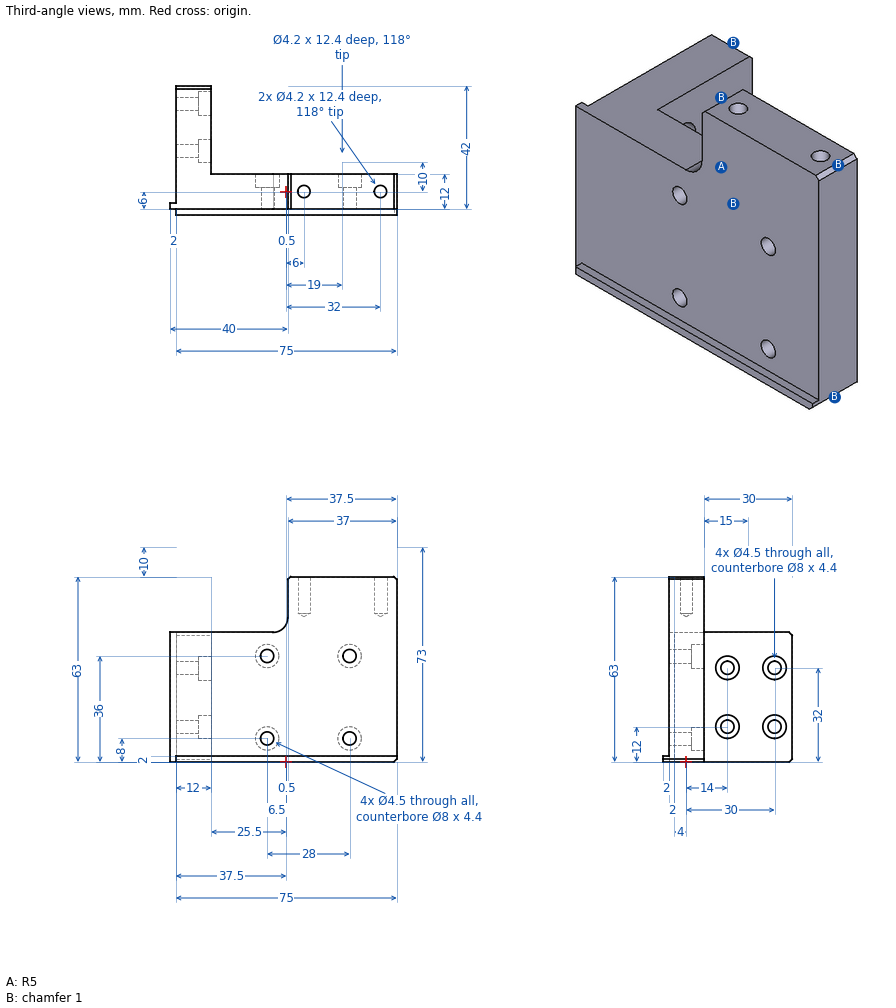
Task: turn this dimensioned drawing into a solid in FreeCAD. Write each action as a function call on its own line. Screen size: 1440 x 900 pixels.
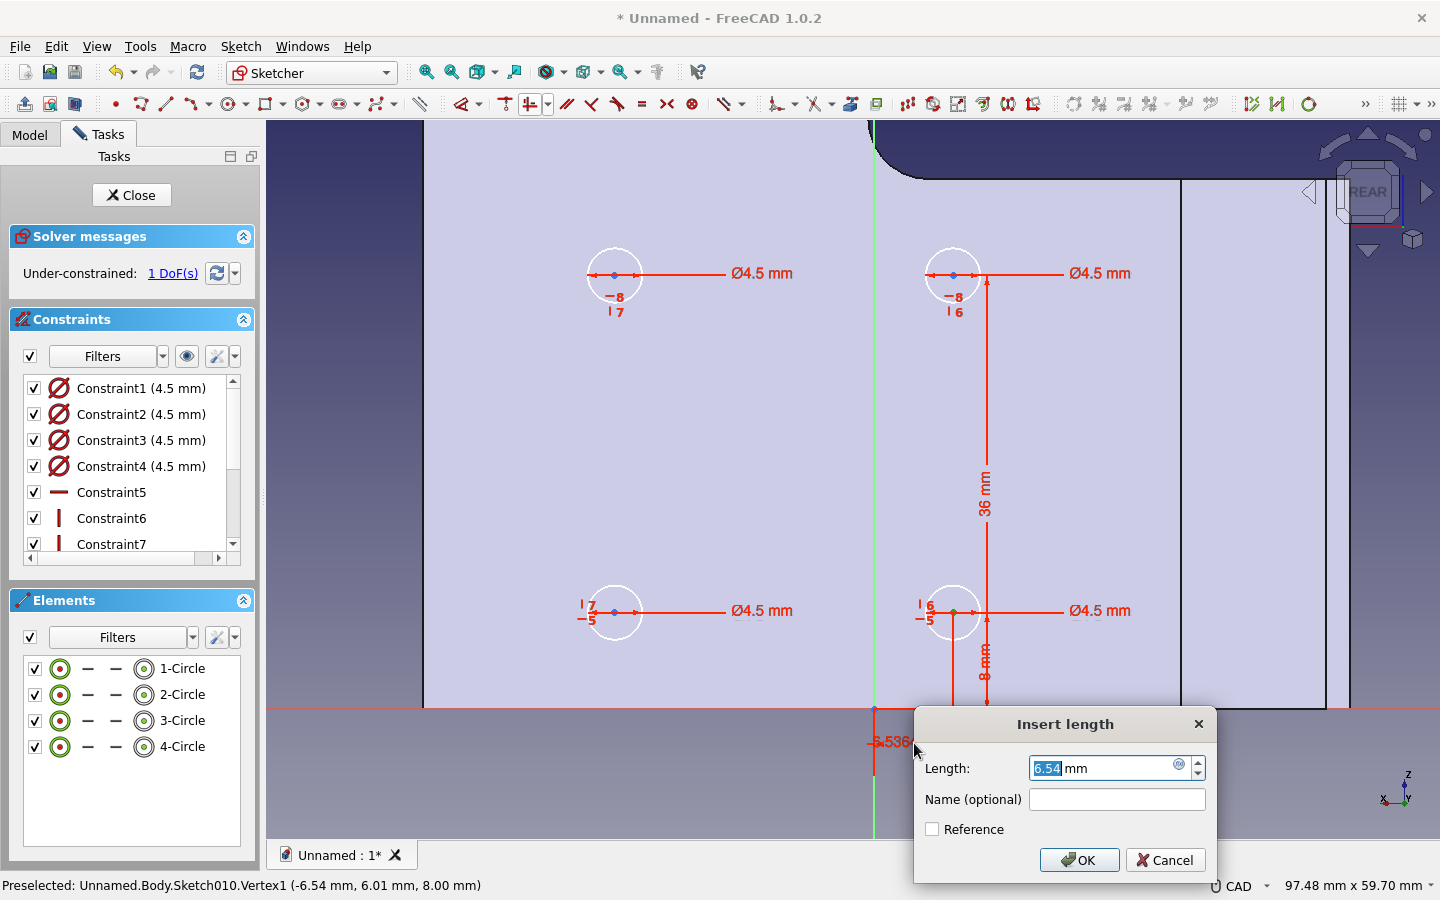
text(6.5)
key(Return)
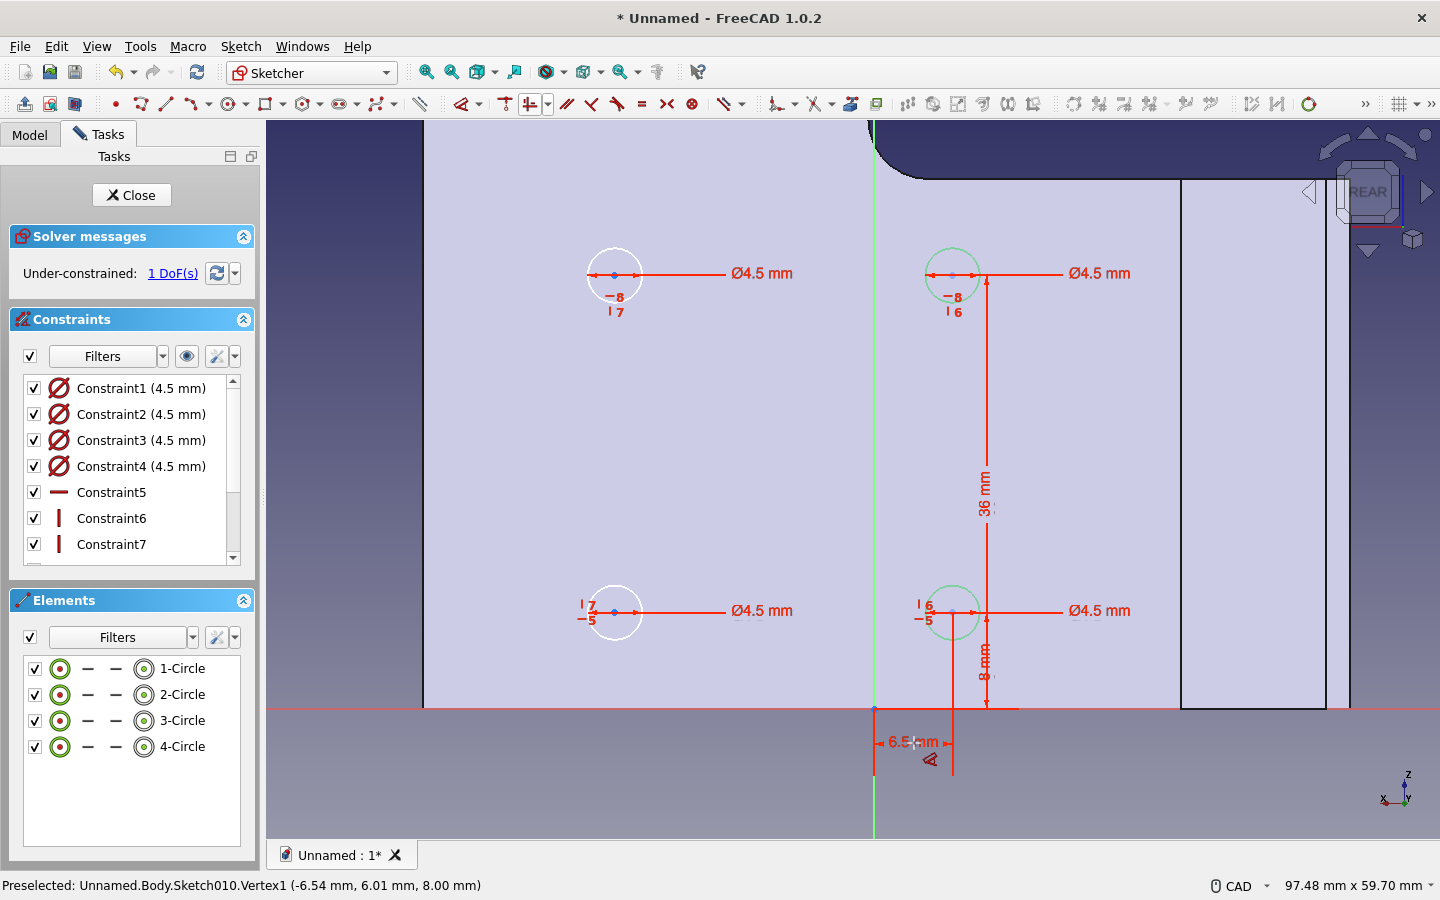
click(953, 613)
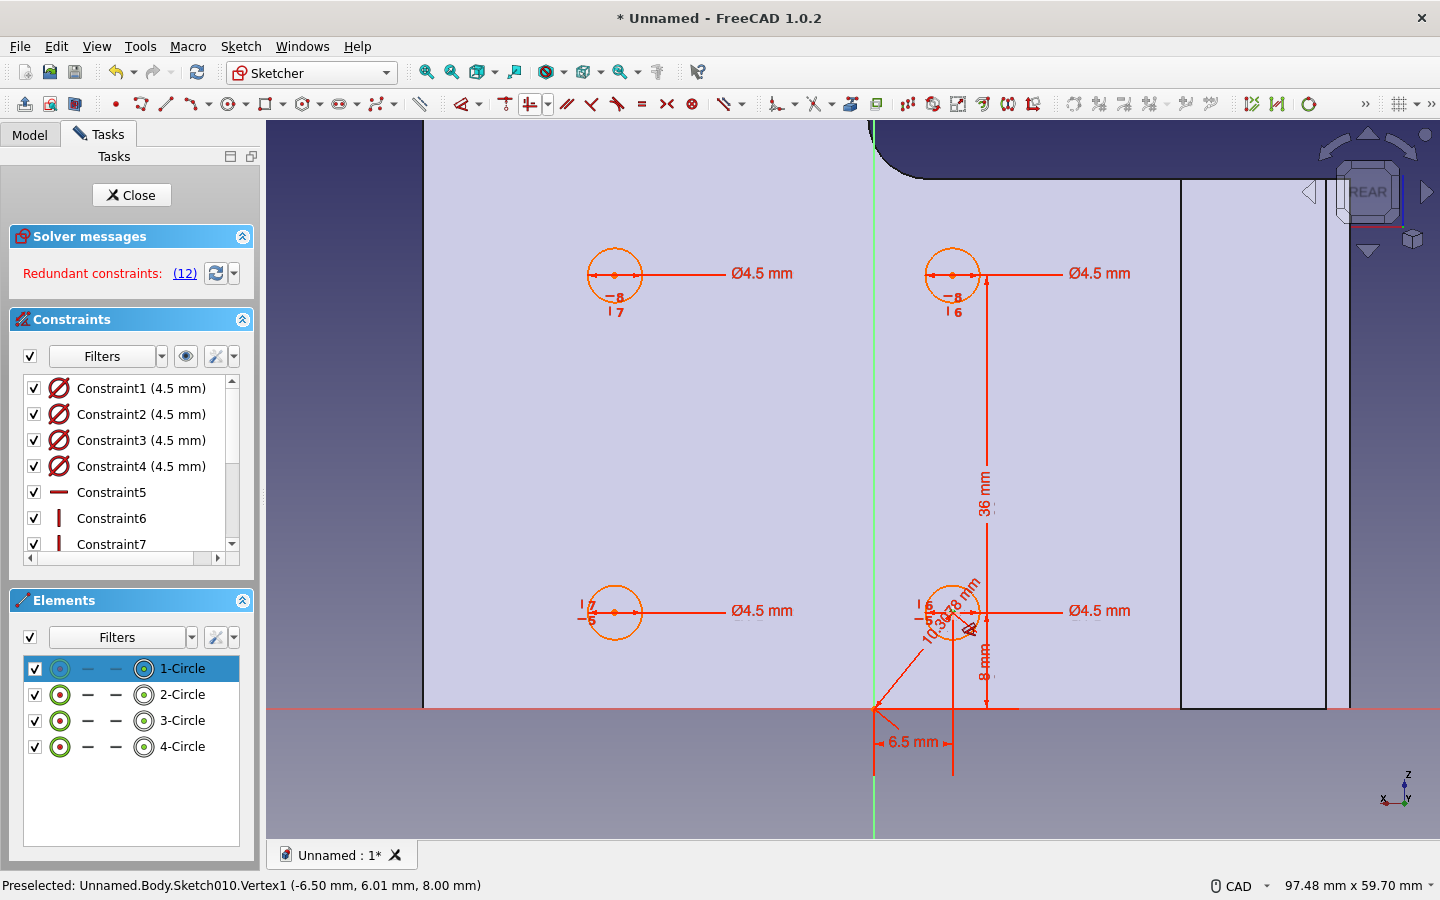
click(615, 613)
click(784, 647)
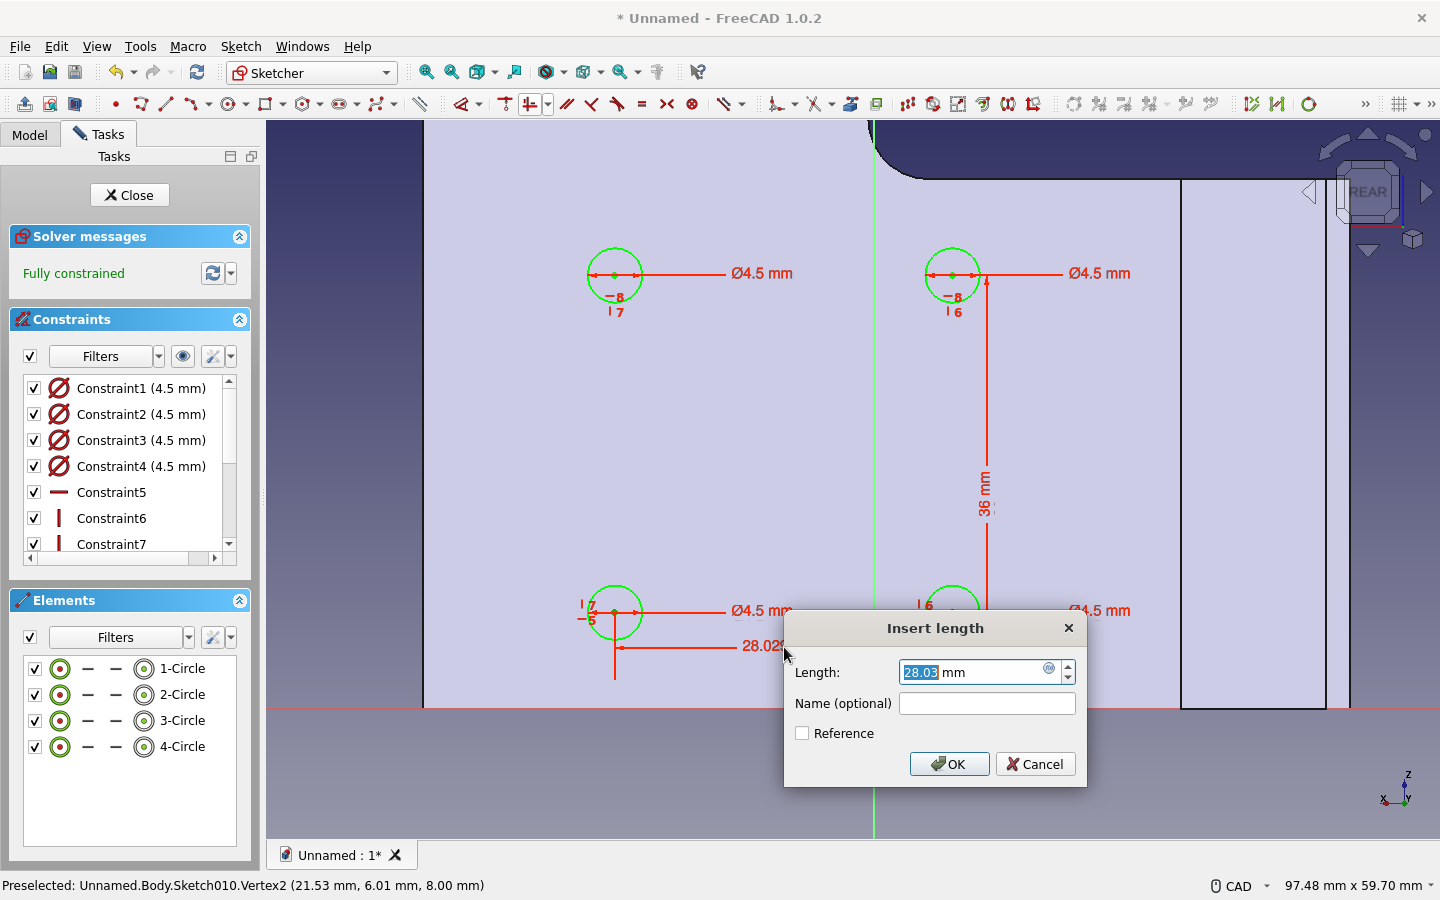
text(28)
key(Return)
key(Escape)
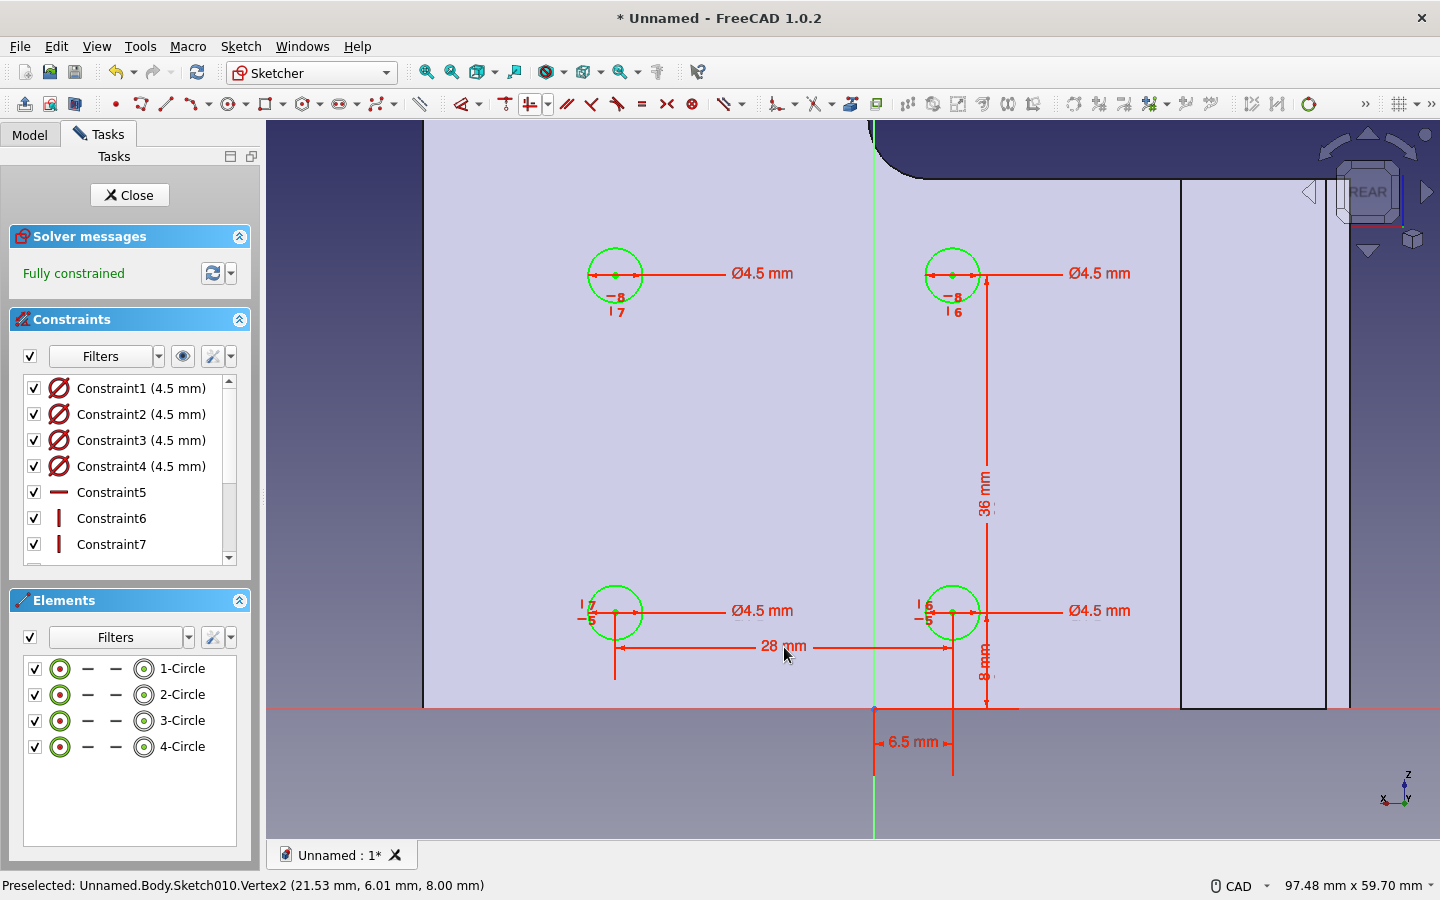
click(130, 195)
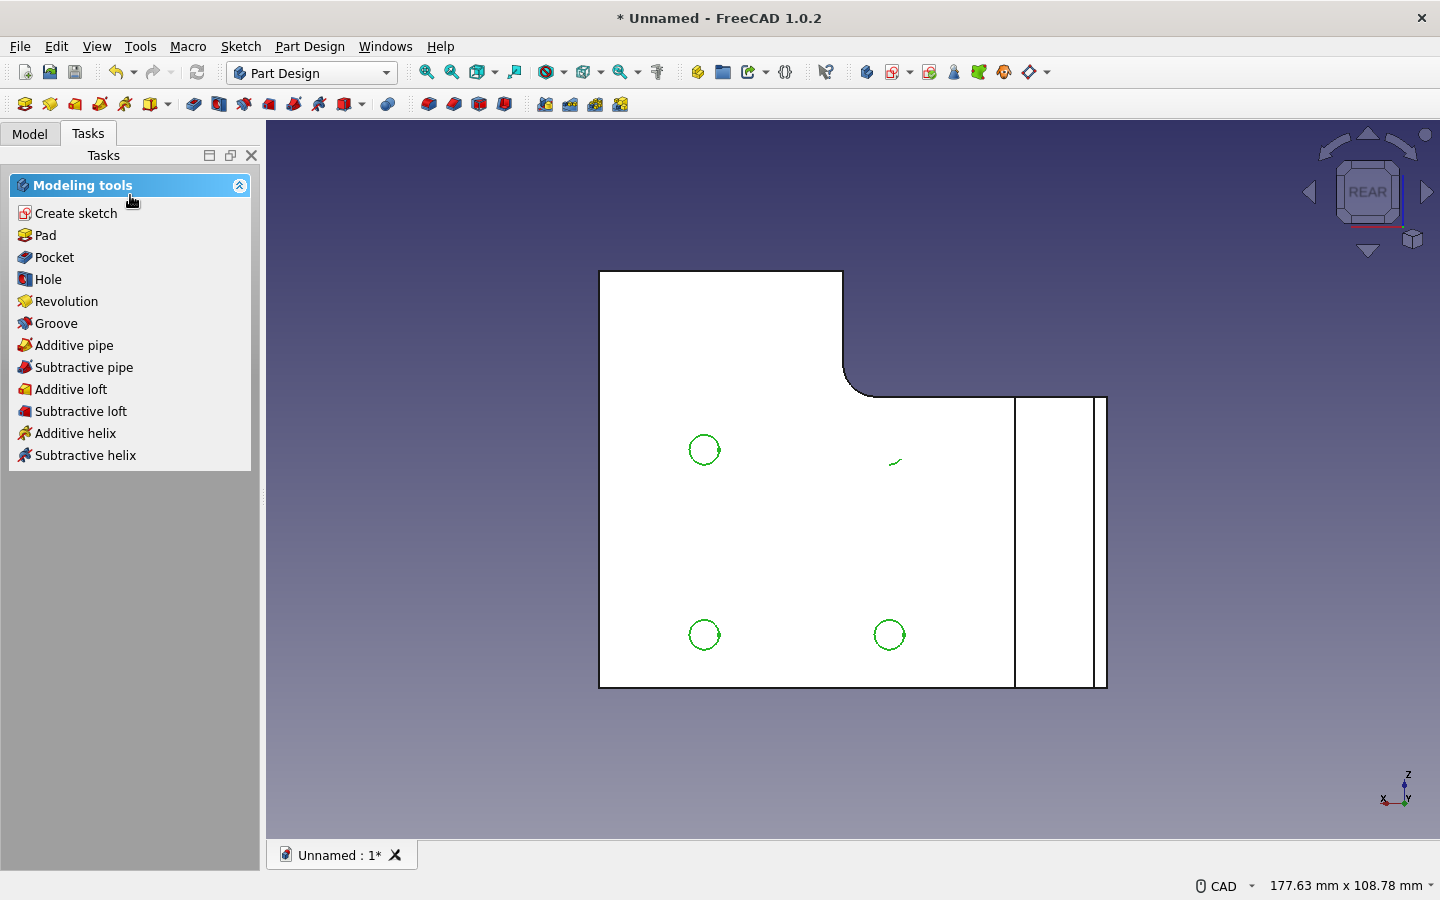
click(219, 104)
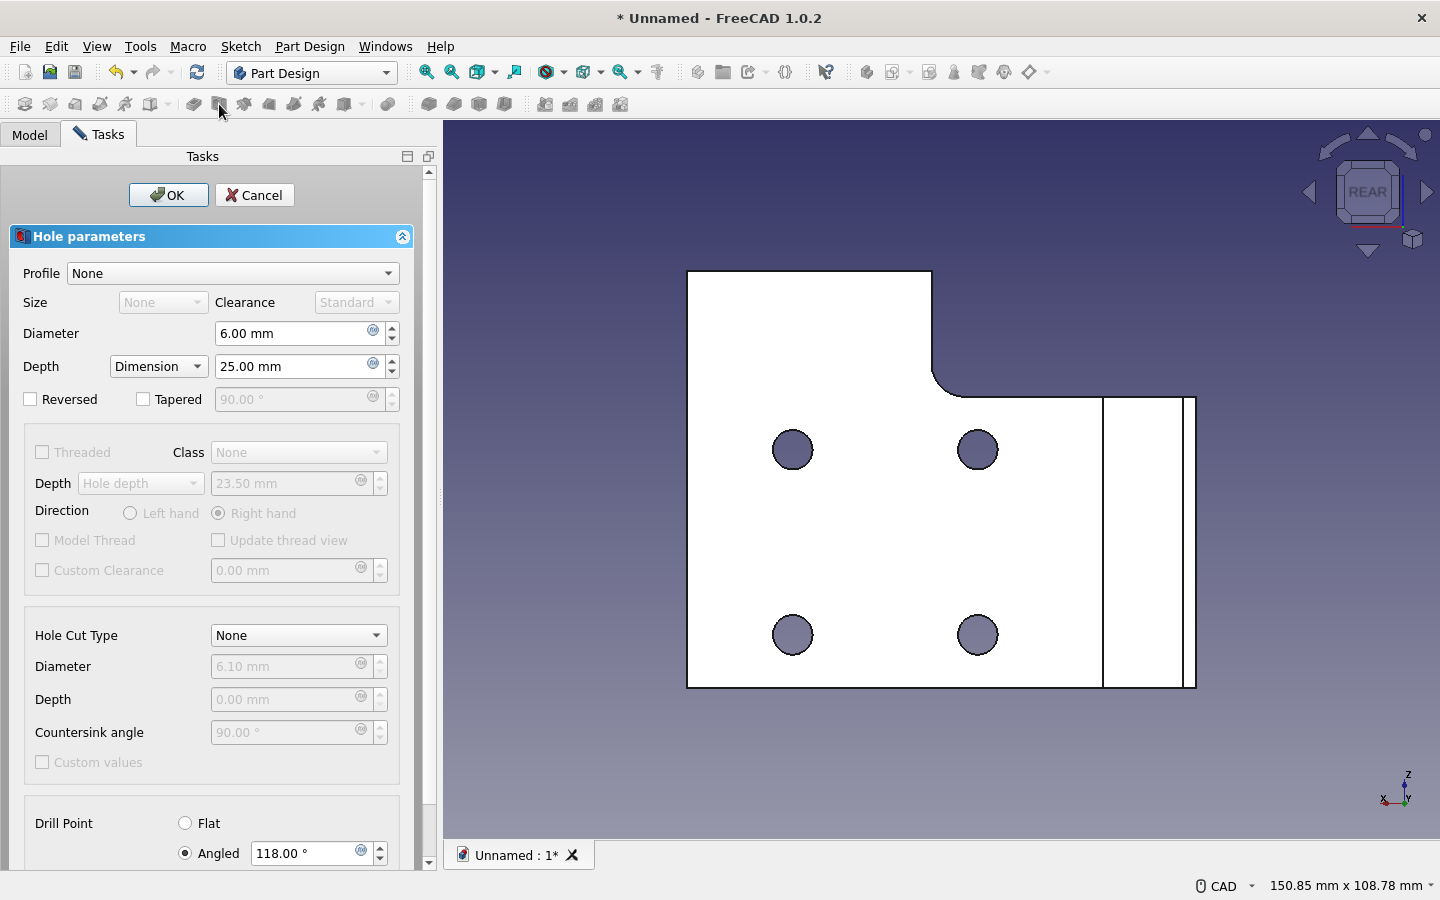
triple_click(300, 334)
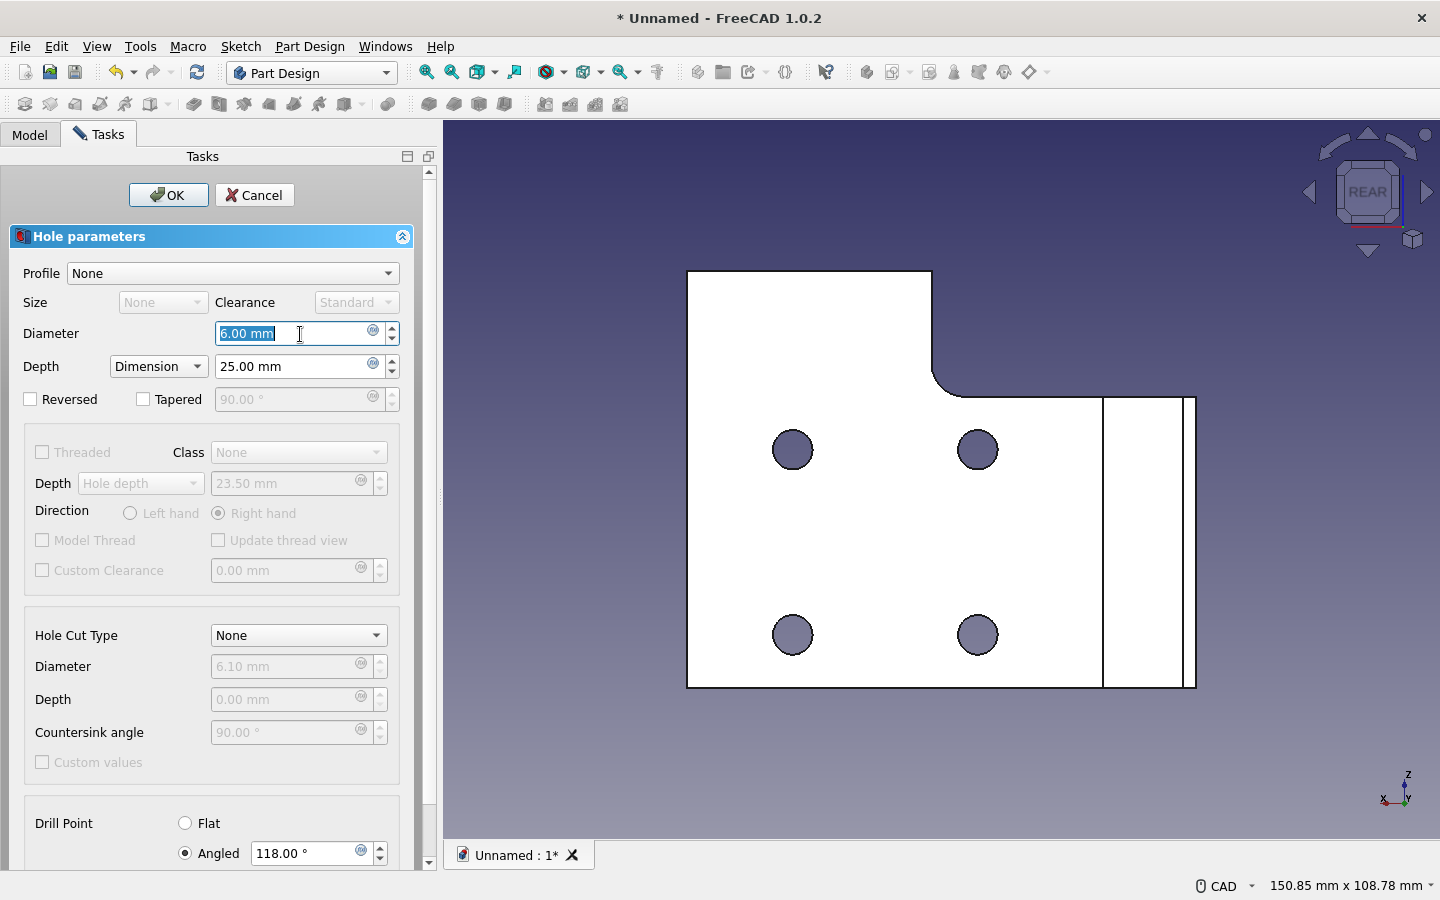
text(4.5)
key(Tab)